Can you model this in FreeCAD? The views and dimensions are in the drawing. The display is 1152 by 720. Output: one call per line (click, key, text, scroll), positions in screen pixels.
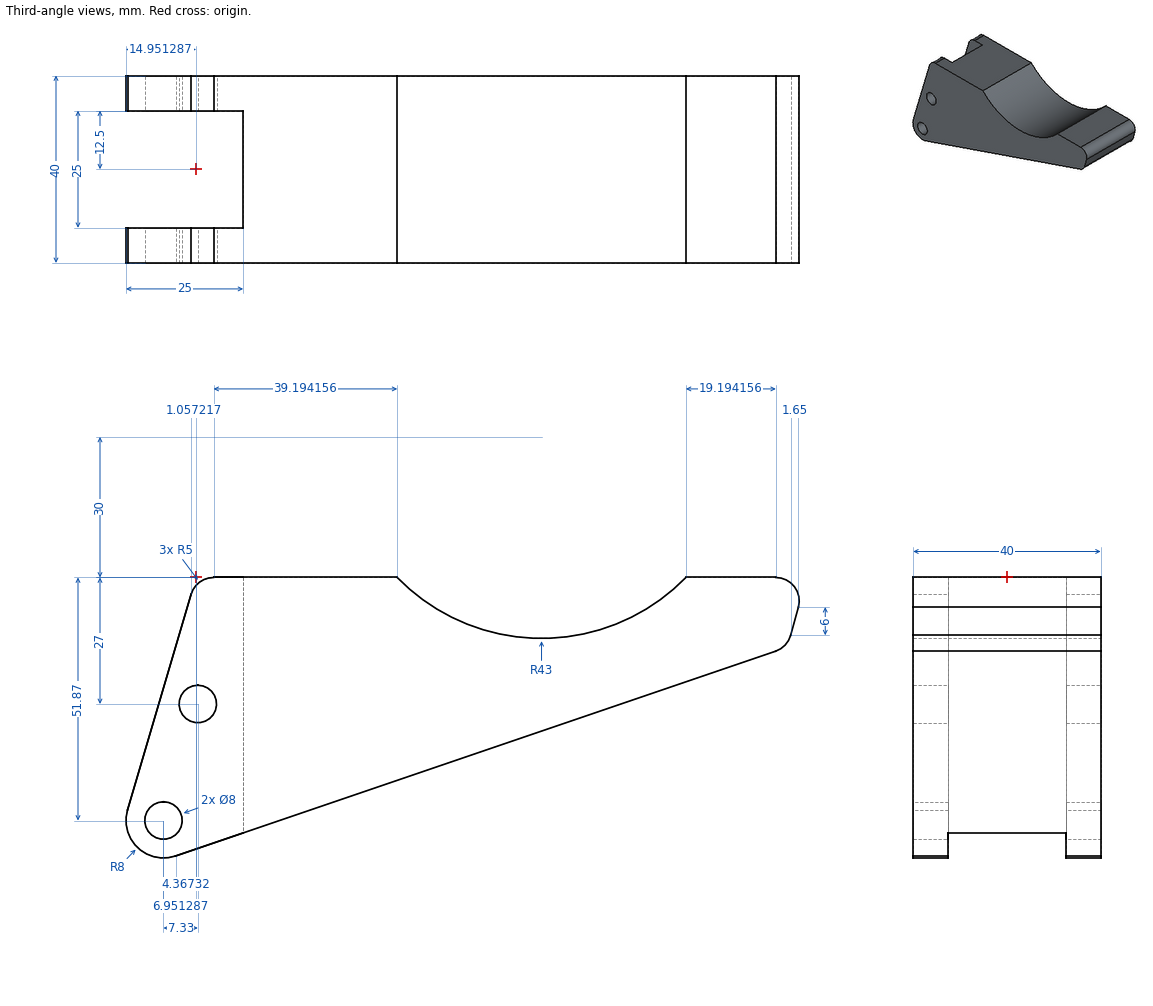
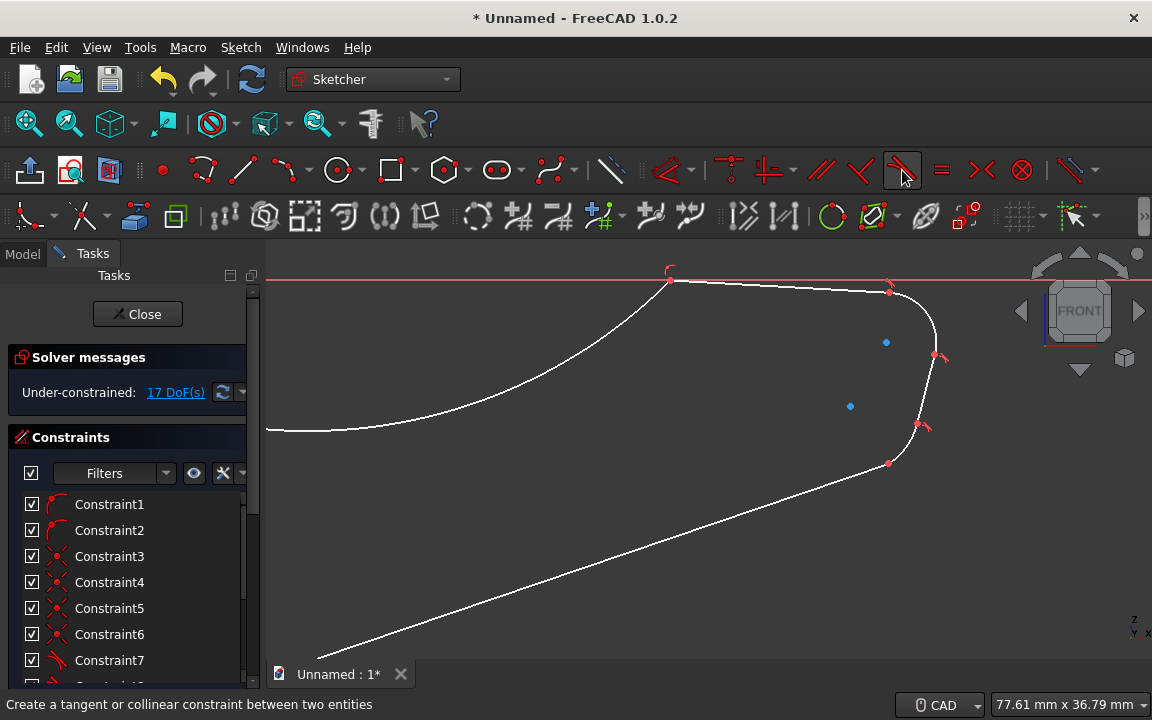
scroll(862, 375, down, 6)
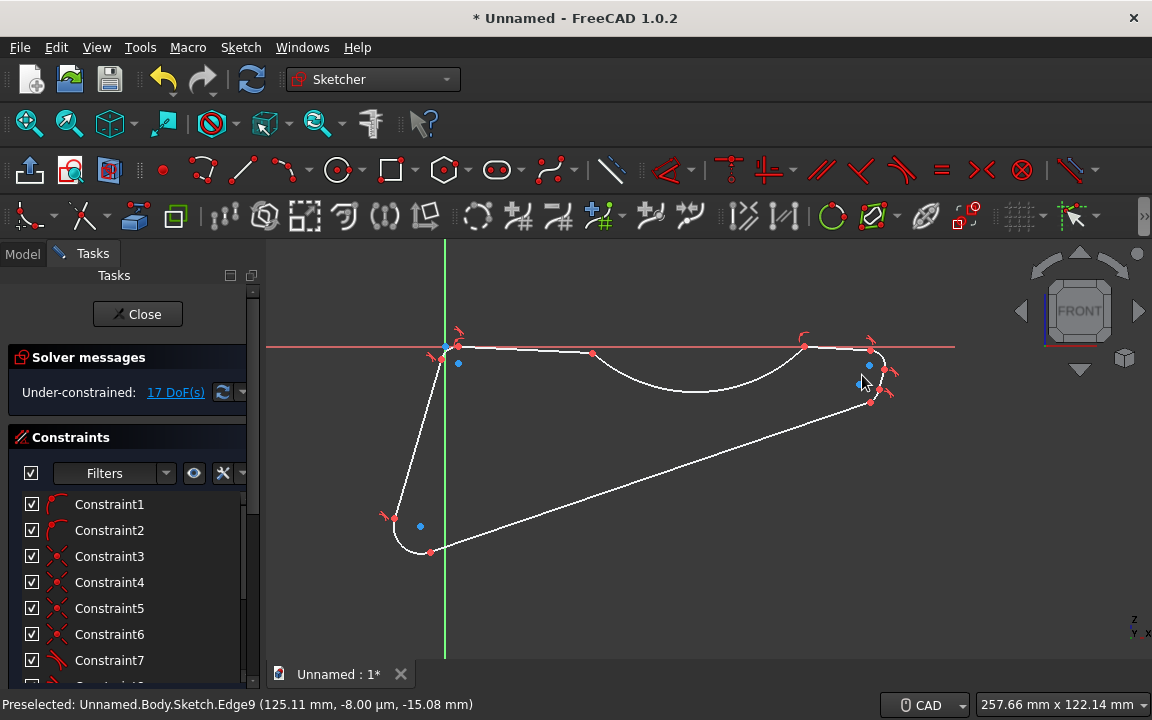
click(738, 447)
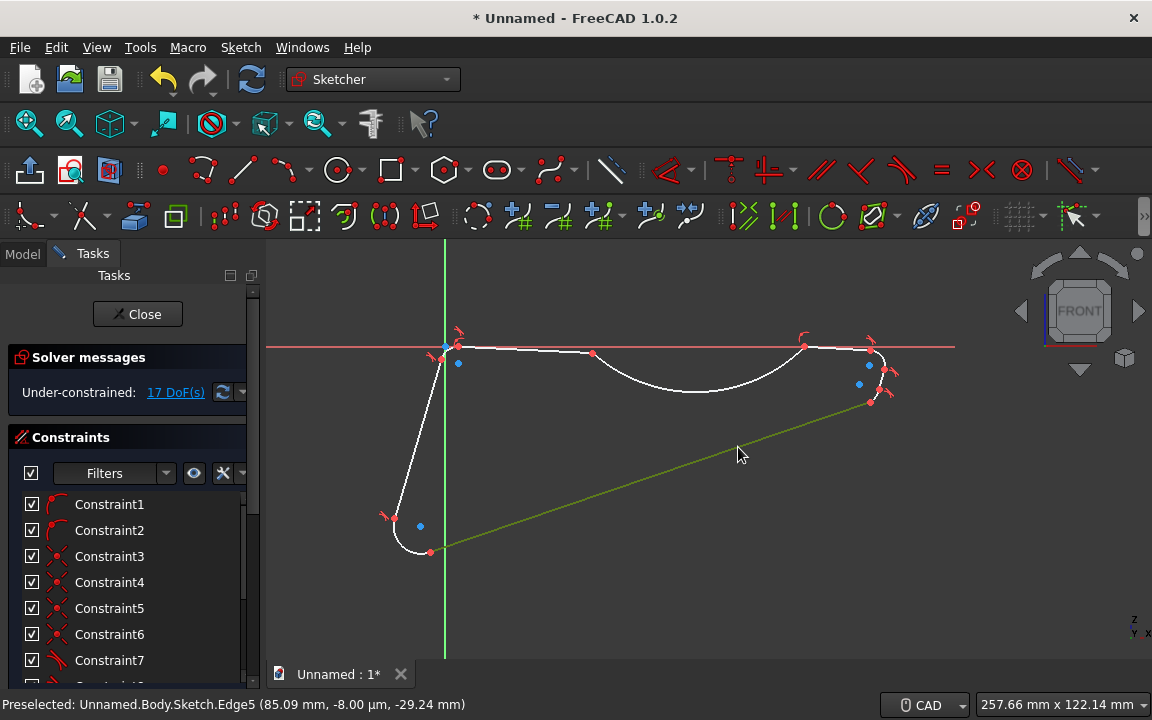
scroll(876, 397, up, 4)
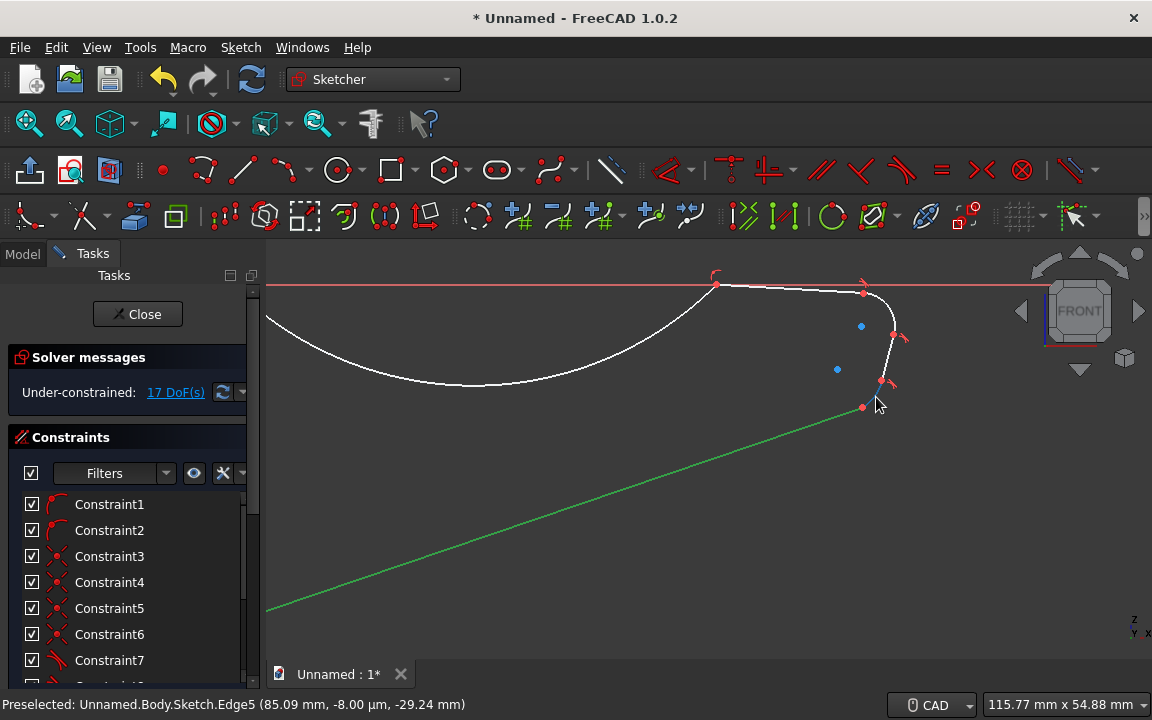
click(875, 396)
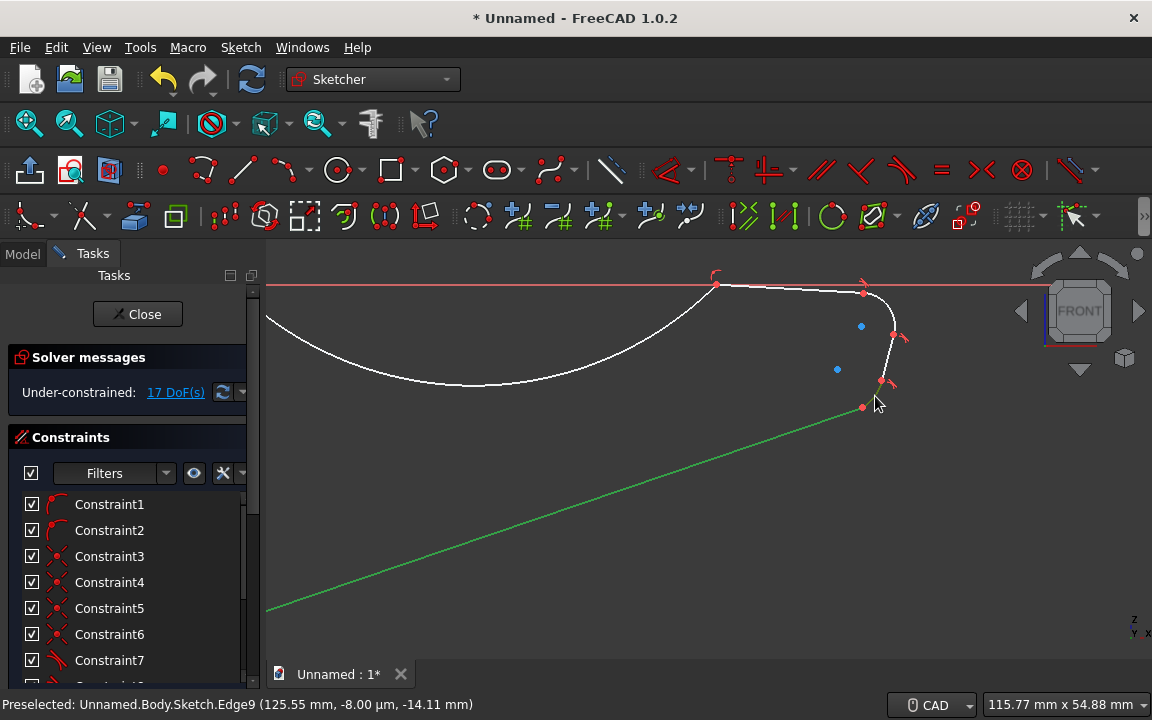
click(902, 170)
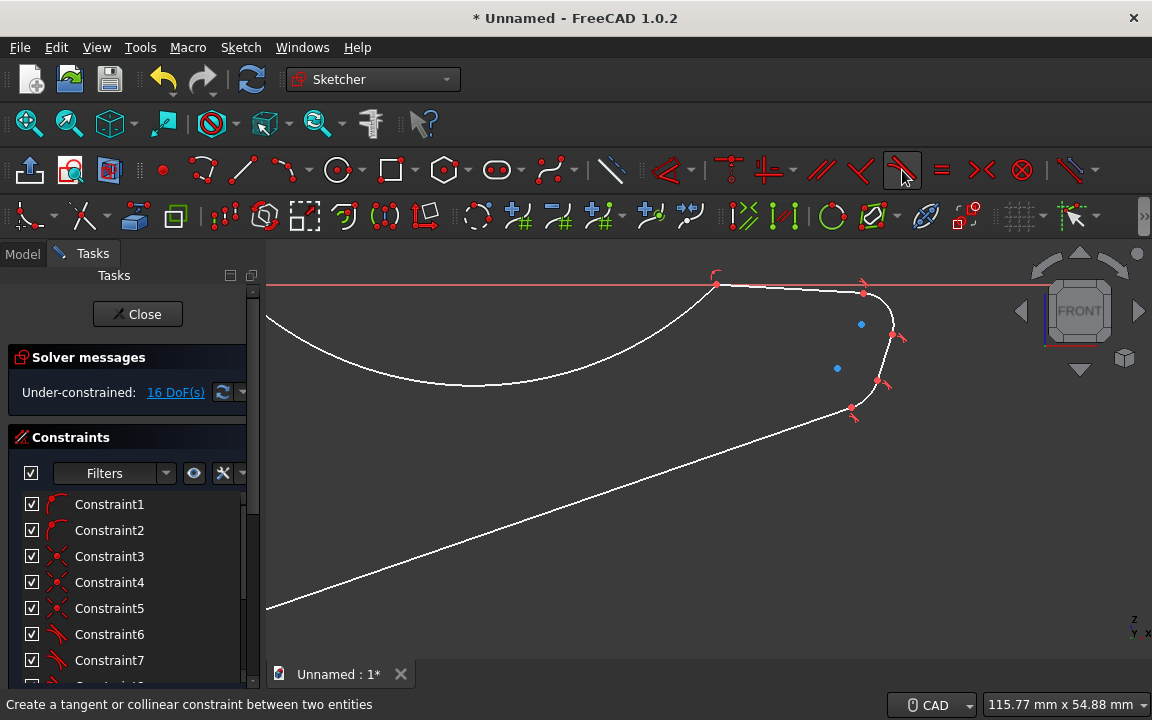
click(561, 508)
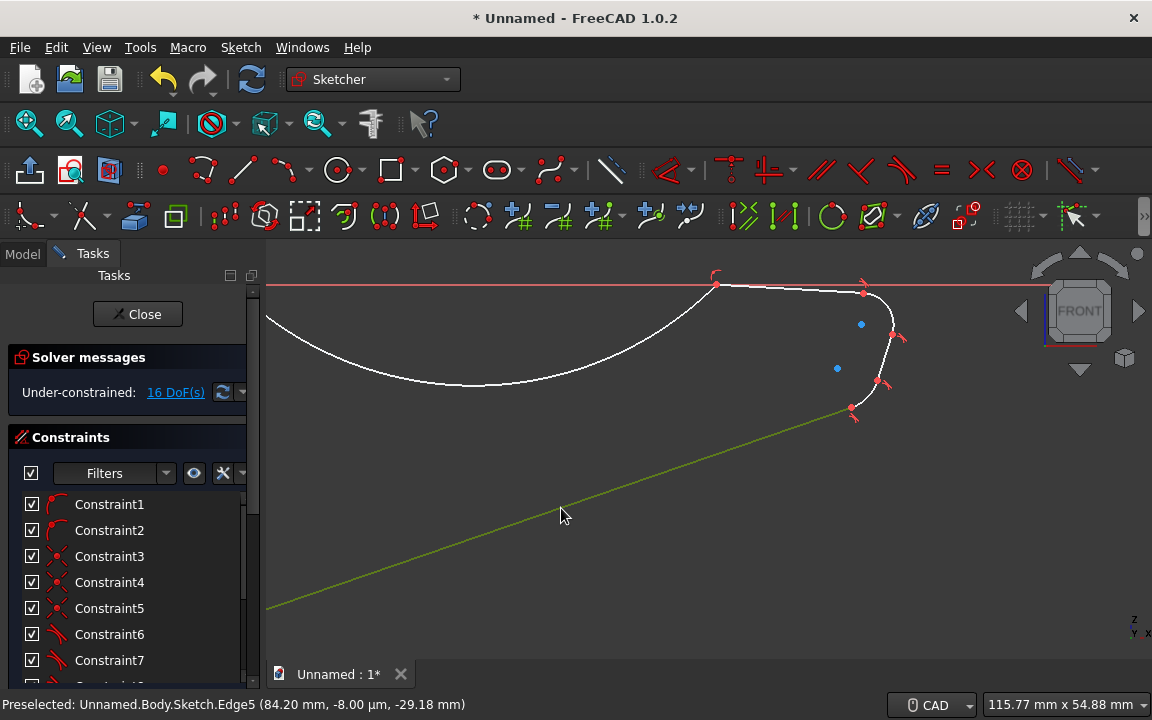
scroll(876, 397, down, 4)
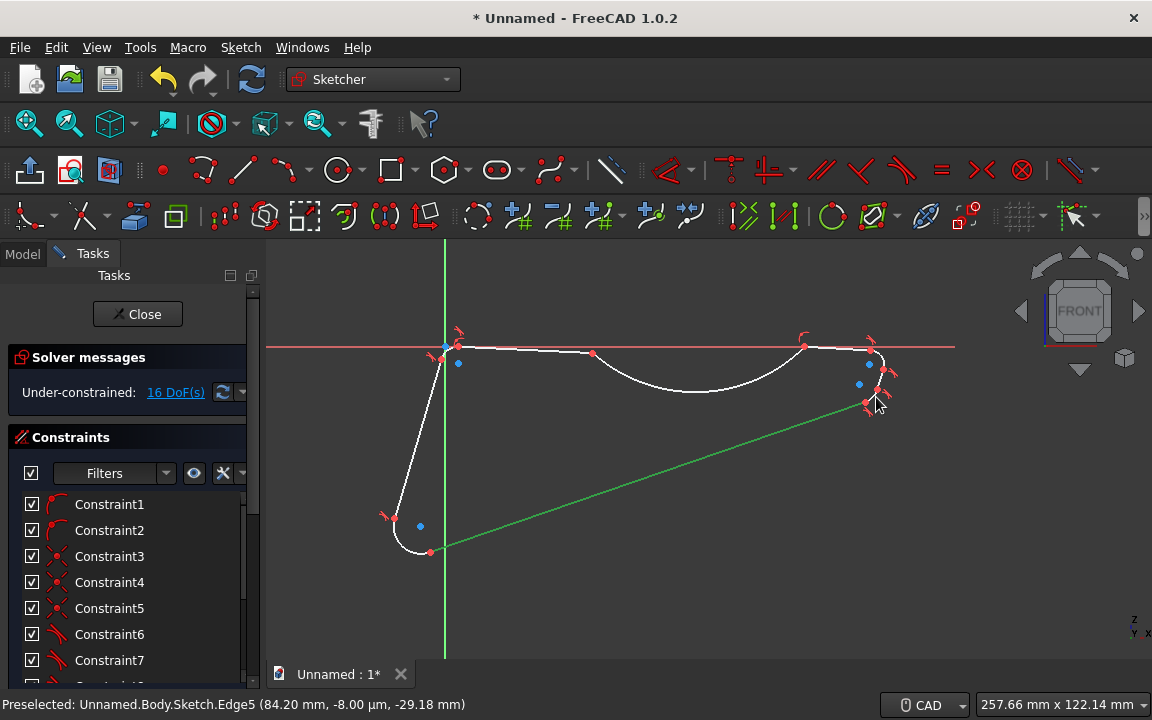
click(396, 537)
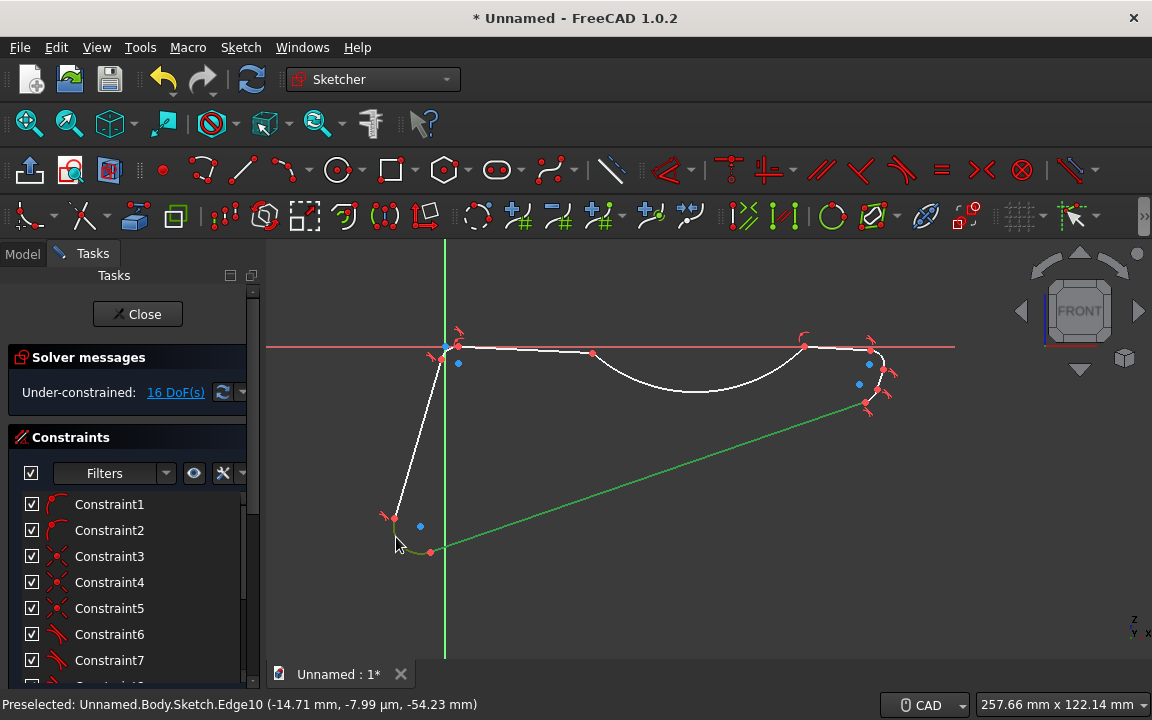
click(902, 170)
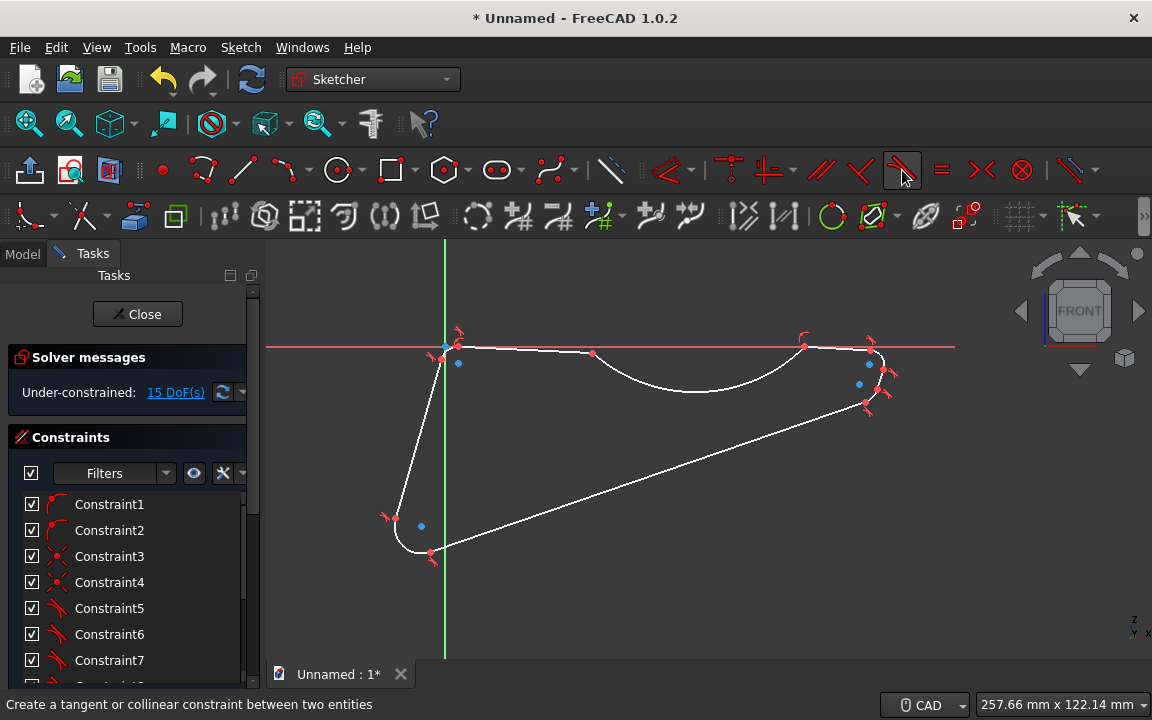
click(499, 349)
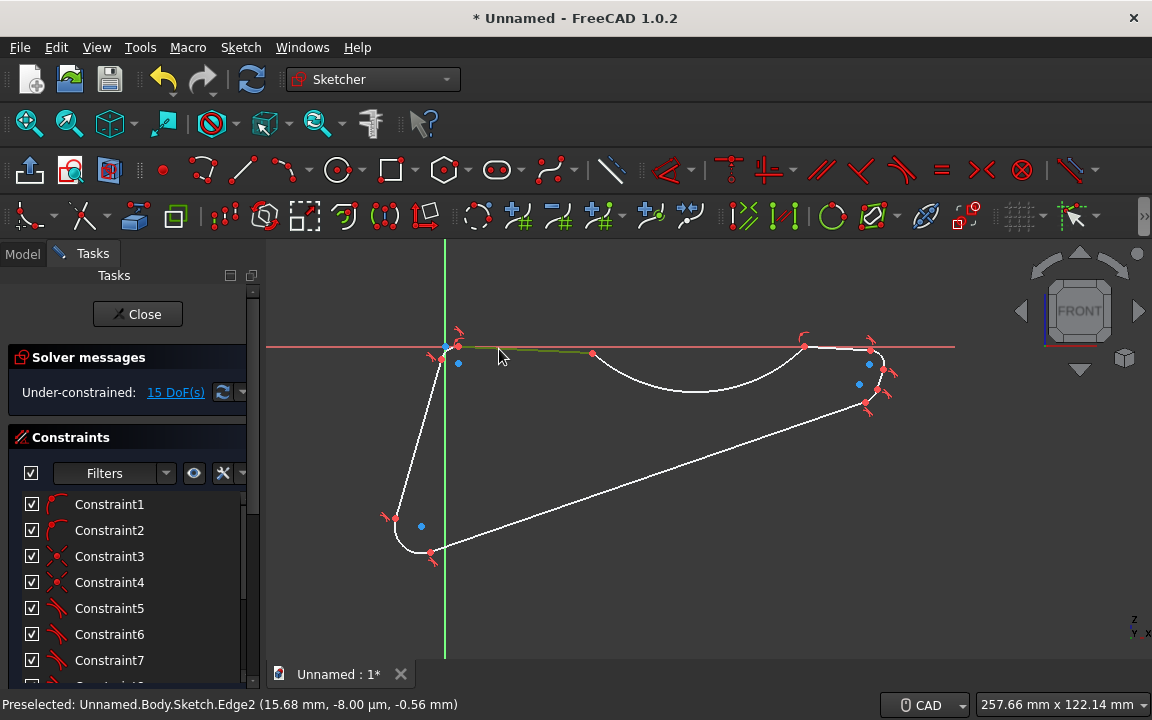
key(h)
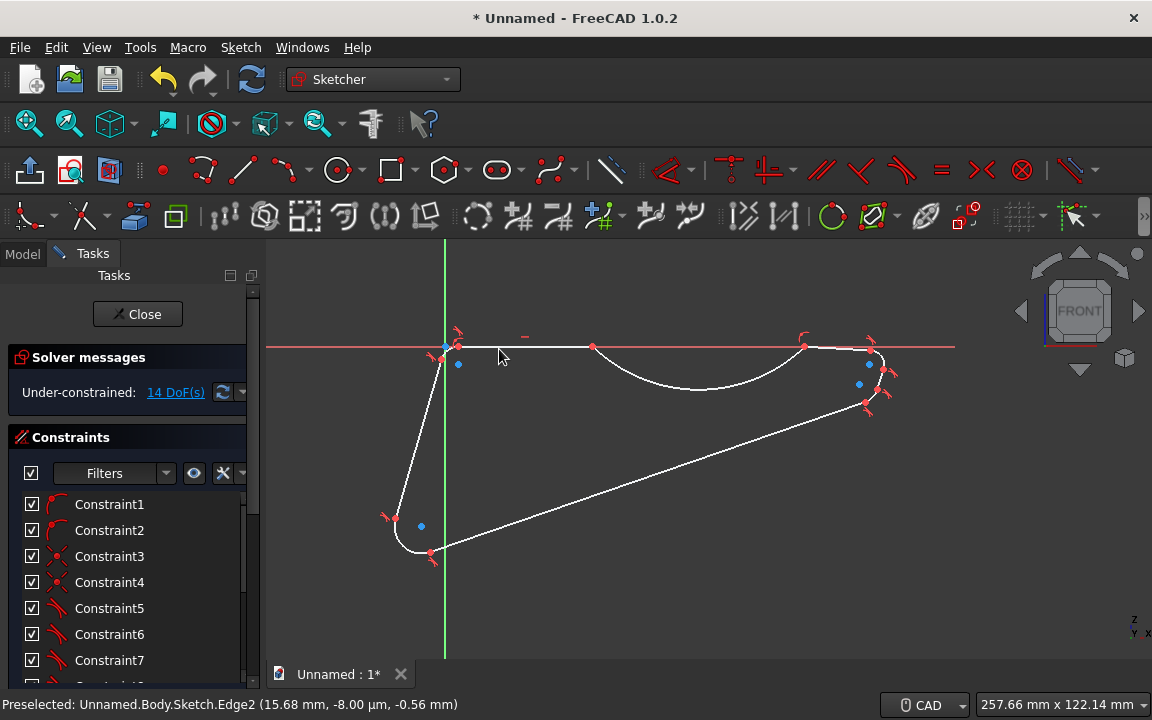
click(825, 348)